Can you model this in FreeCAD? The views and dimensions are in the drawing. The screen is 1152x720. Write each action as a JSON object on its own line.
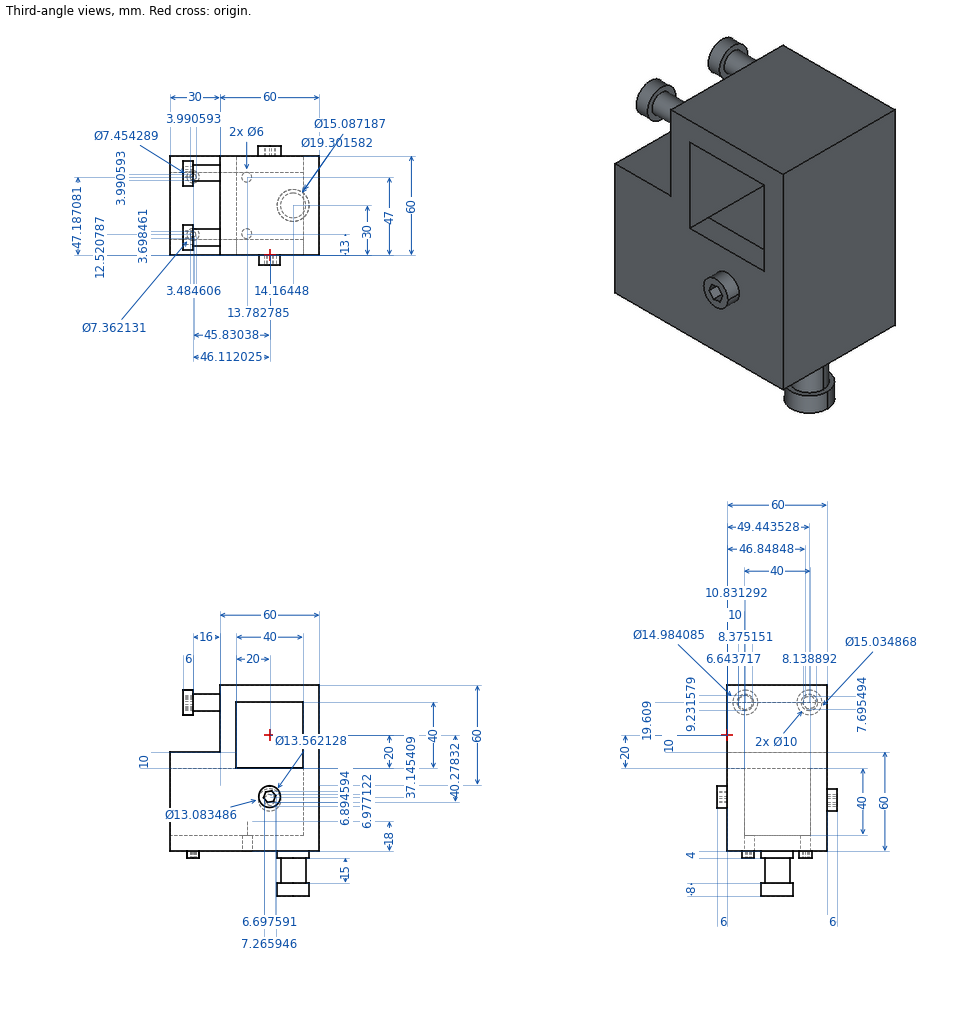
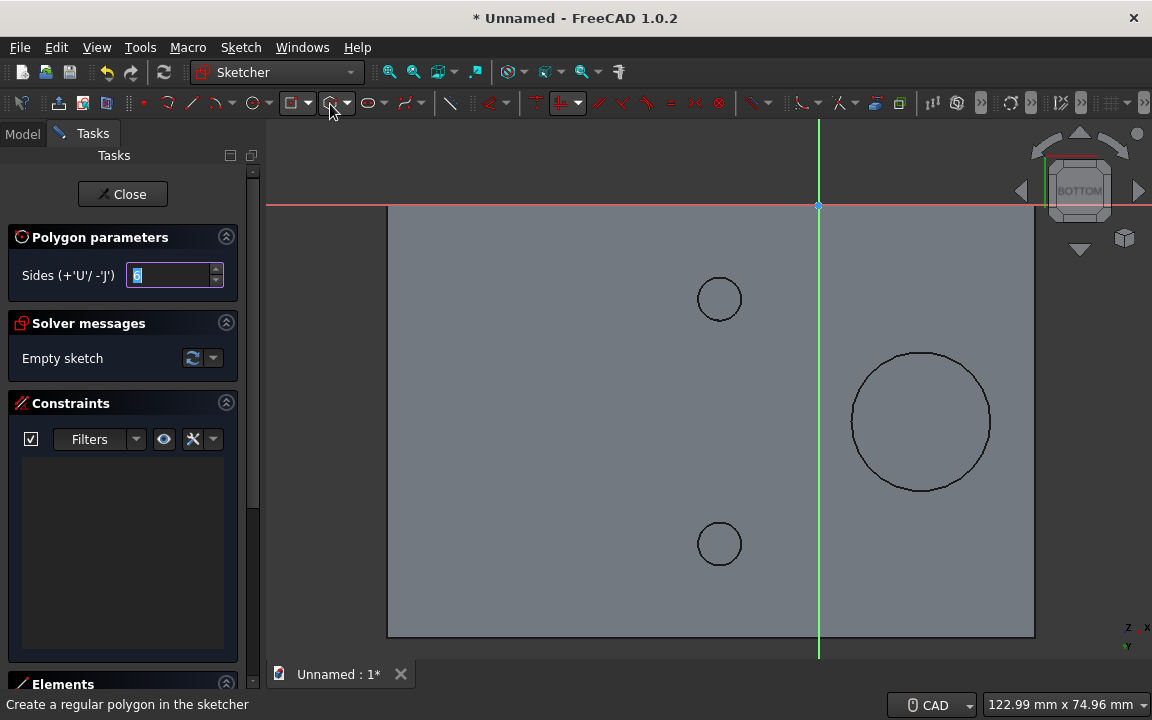
{"action": "scroll", "coordinate": [487, 545], "scroll_direction": "up", "scroll_amount": 4}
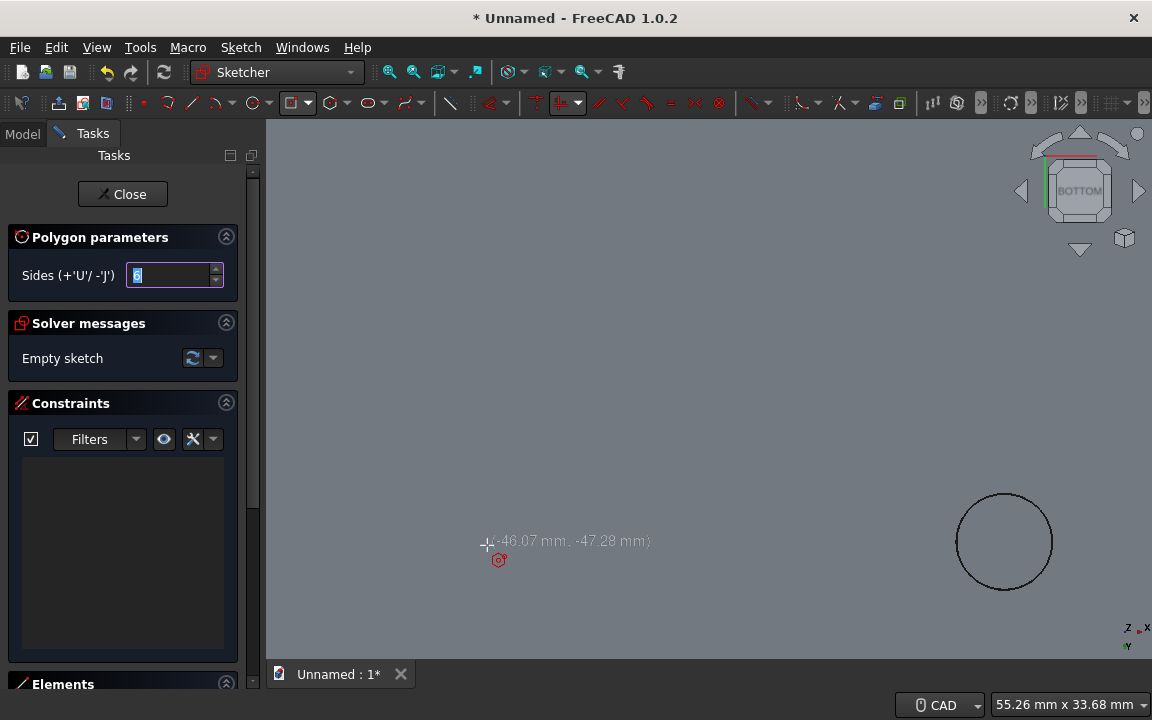
{"action": "left_click", "coordinate": [486, 545]}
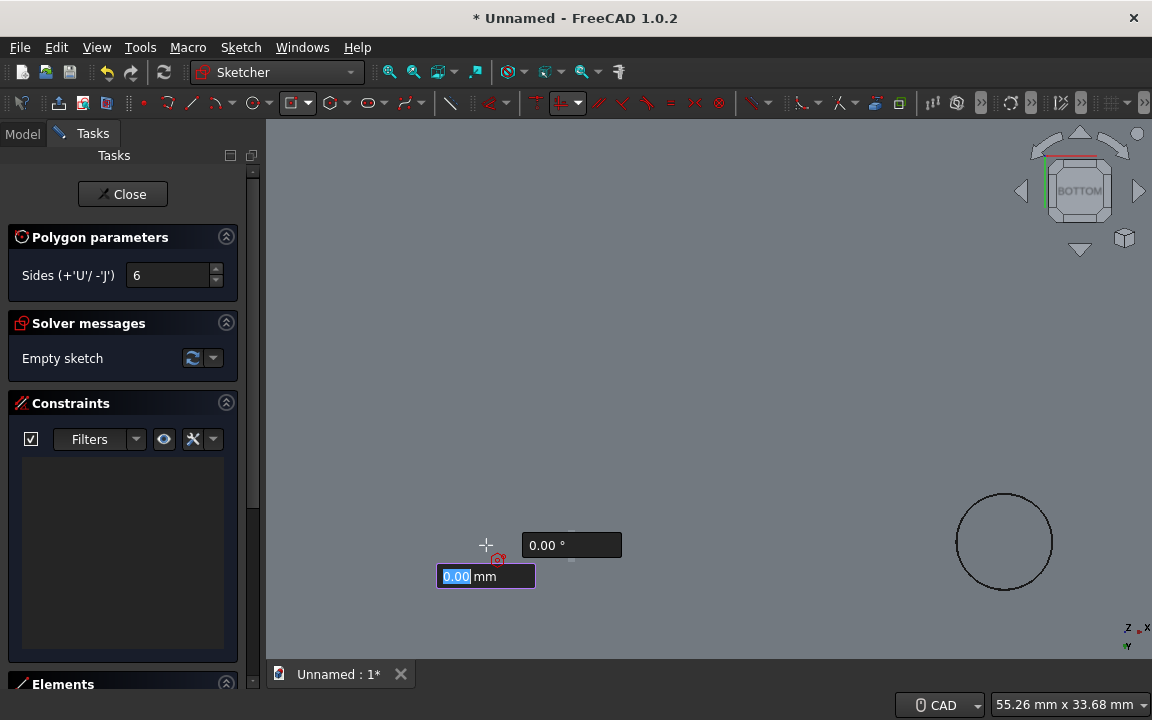
{"action": "left_click", "coordinate": [454, 553]}
{"action": "right_click", "coordinate": [454, 553]}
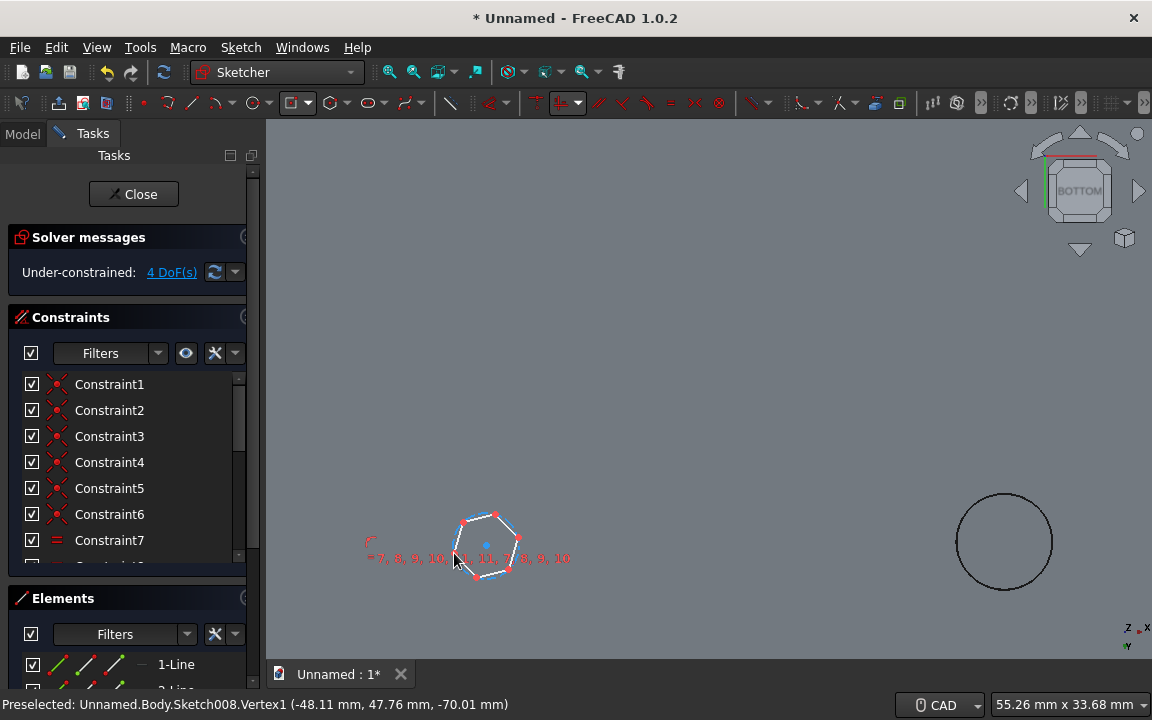
{"action": "left_click", "coordinate": [330, 104]}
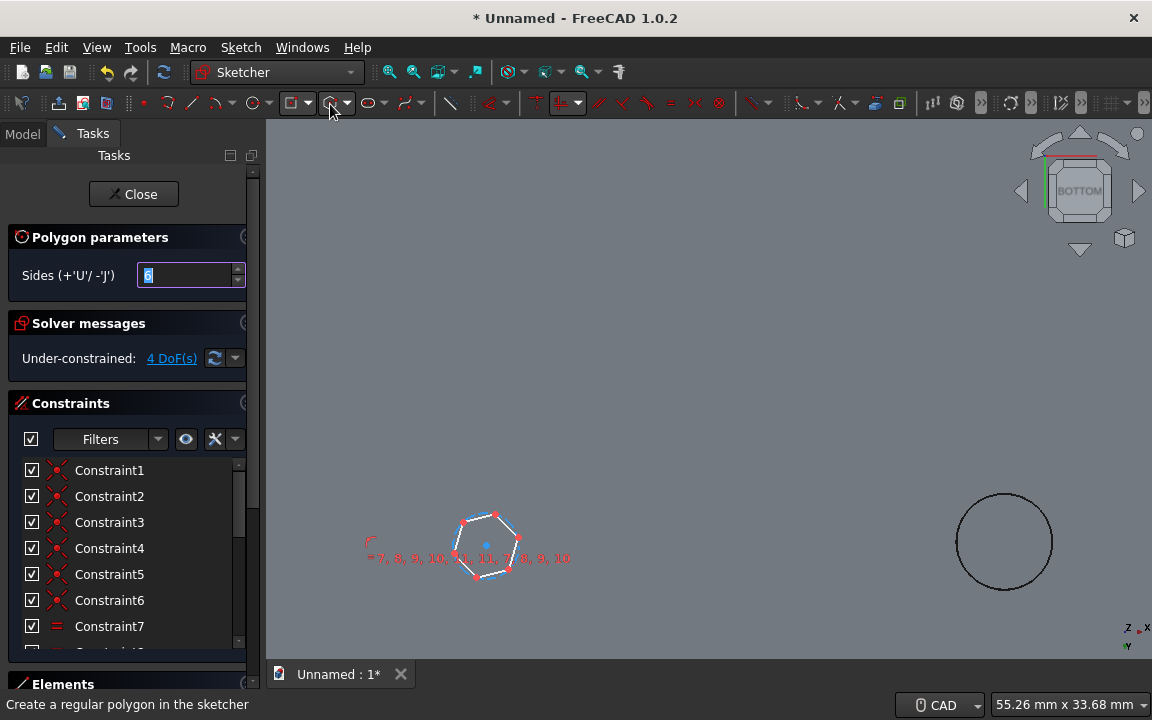
{"action": "scroll", "coordinate": [489, 546], "scroll_direction": "down", "scroll_amount": 4}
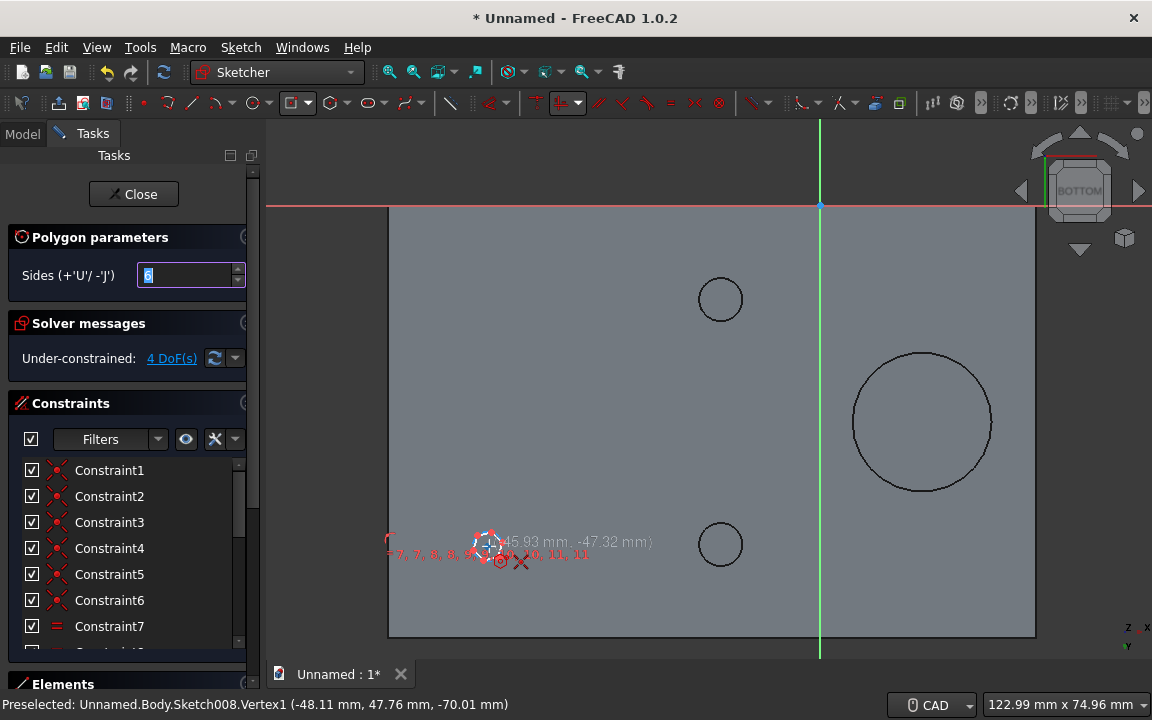
{"action": "scroll", "coordinate": [488, 296], "scroll_direction": "up", "scroll_amount": 5}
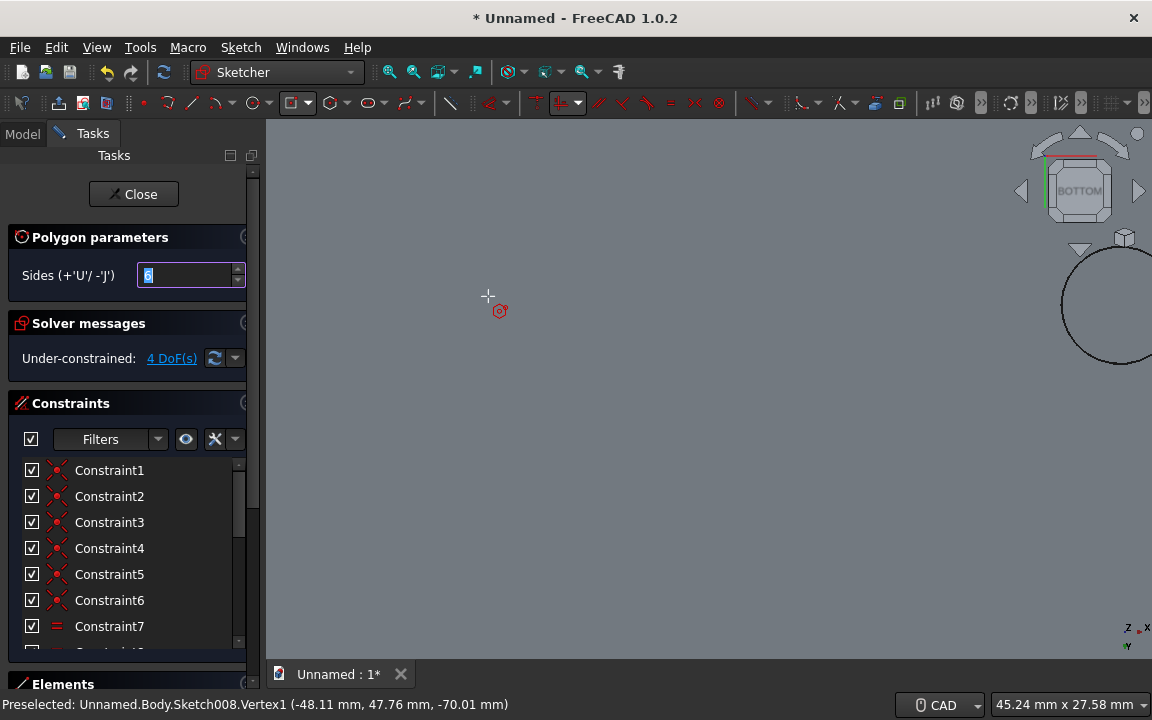
{"action": "left_click", "coordinate": [487, 296]}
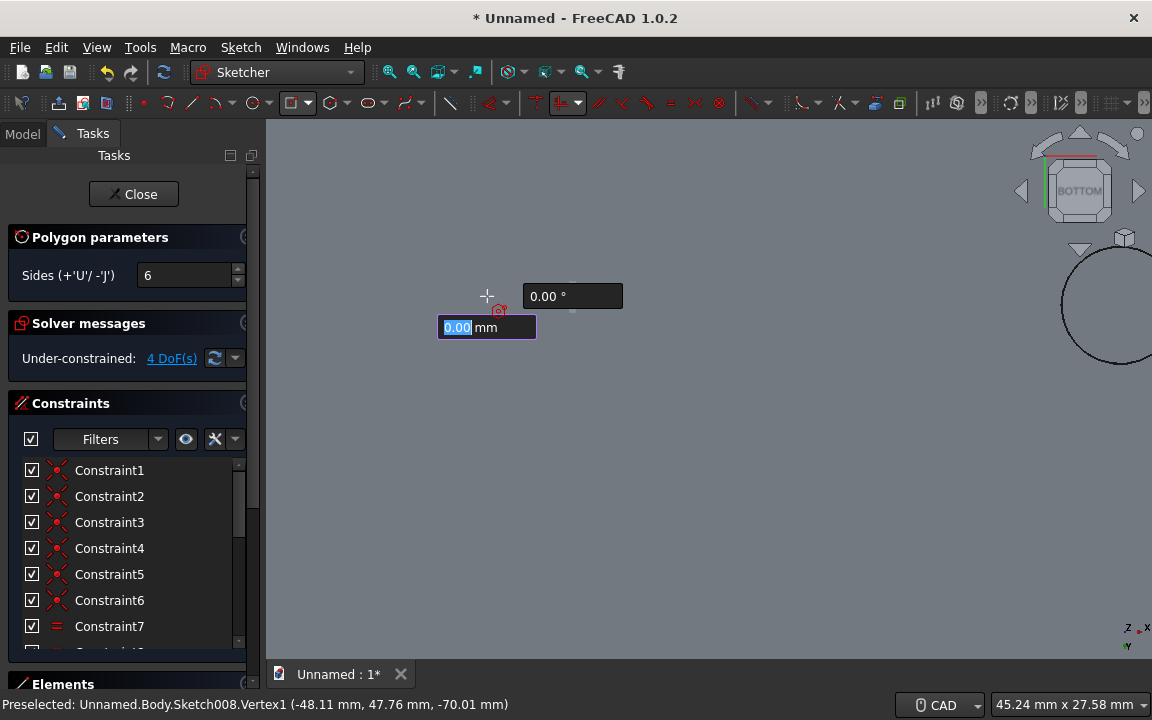
{"action": "left_click", "coordinate": [482, 332]}
{"action": "right_click", "coordinate": [482, 332]}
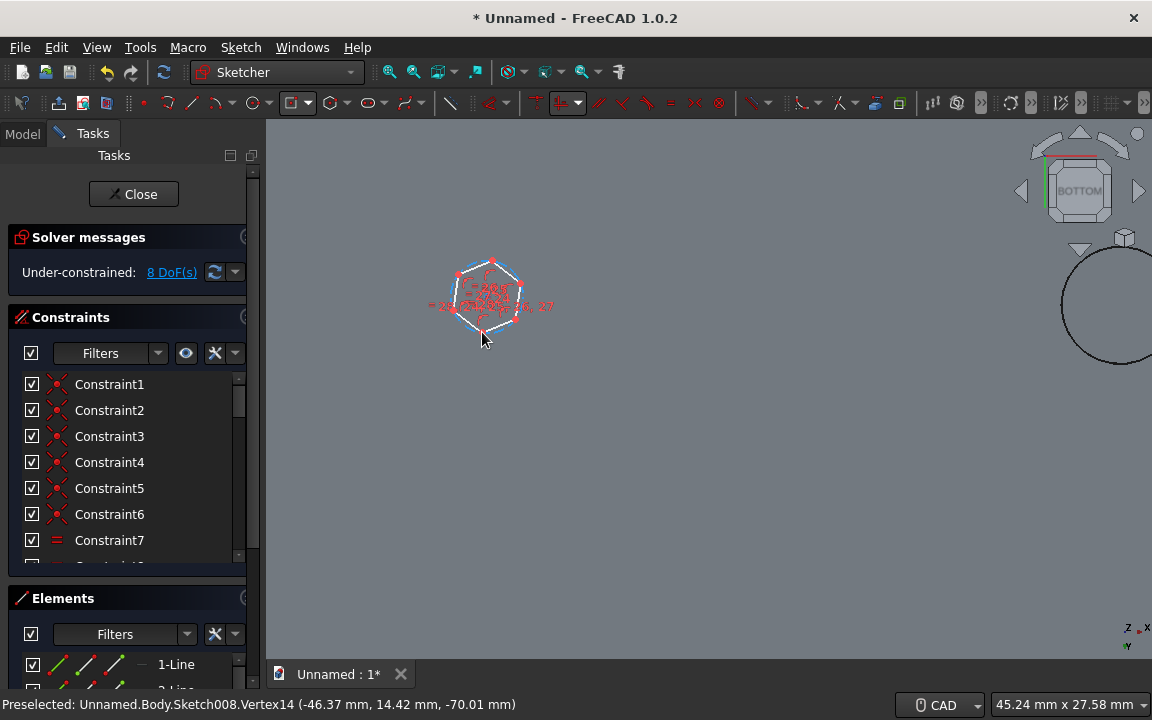
{"action": "left_click", "coordinate": [254, 104]}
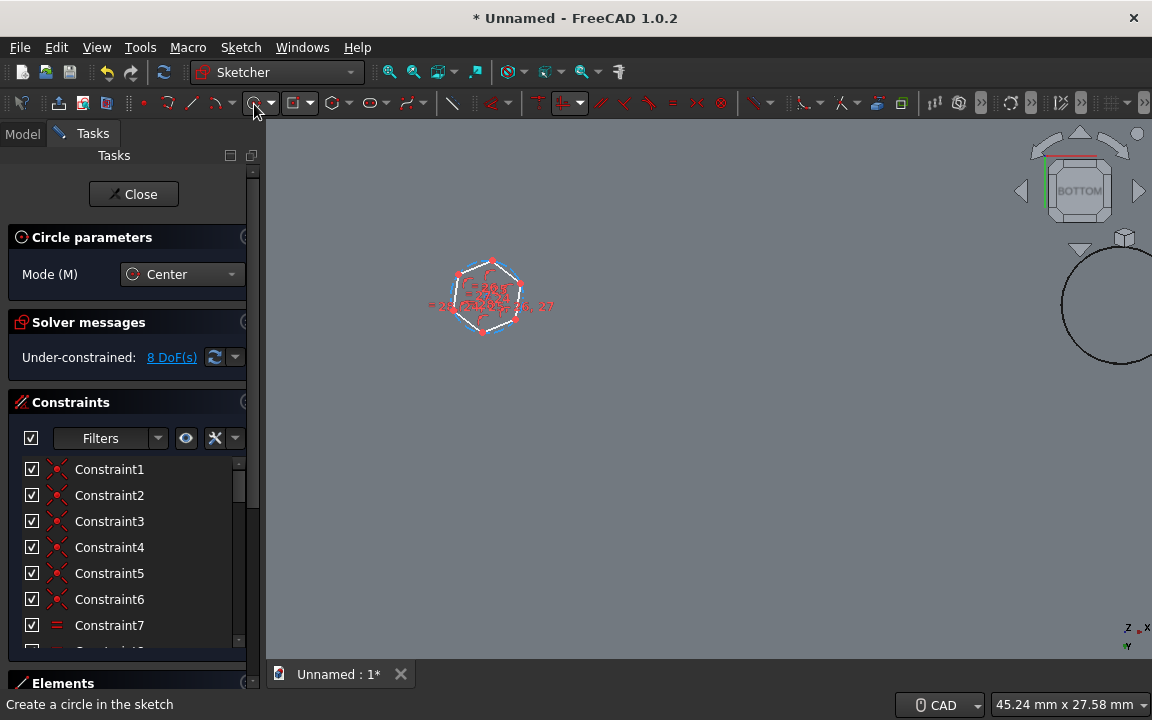
{"action": "scroll", "coordinate": [488, 296], "scroll_direction": "down", "scroll_amount": 5}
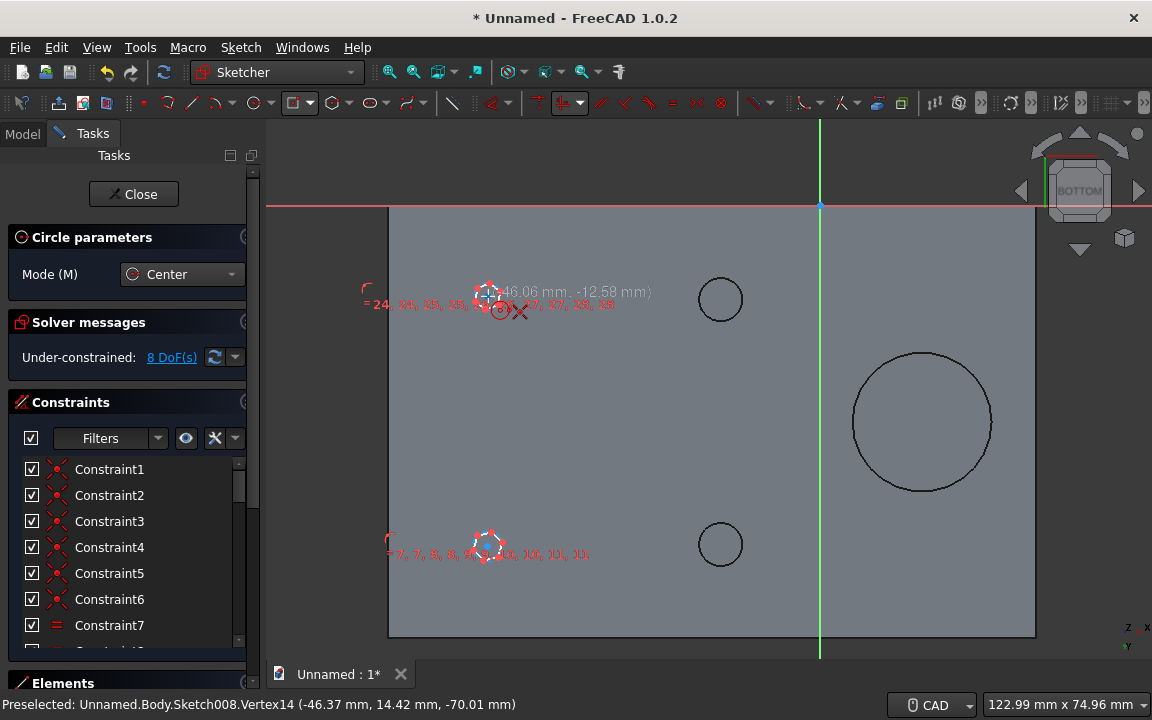
{"action": "scroll", "coordinate": [488, 546], "scroll_direction": "up", "scroll_amount": 2}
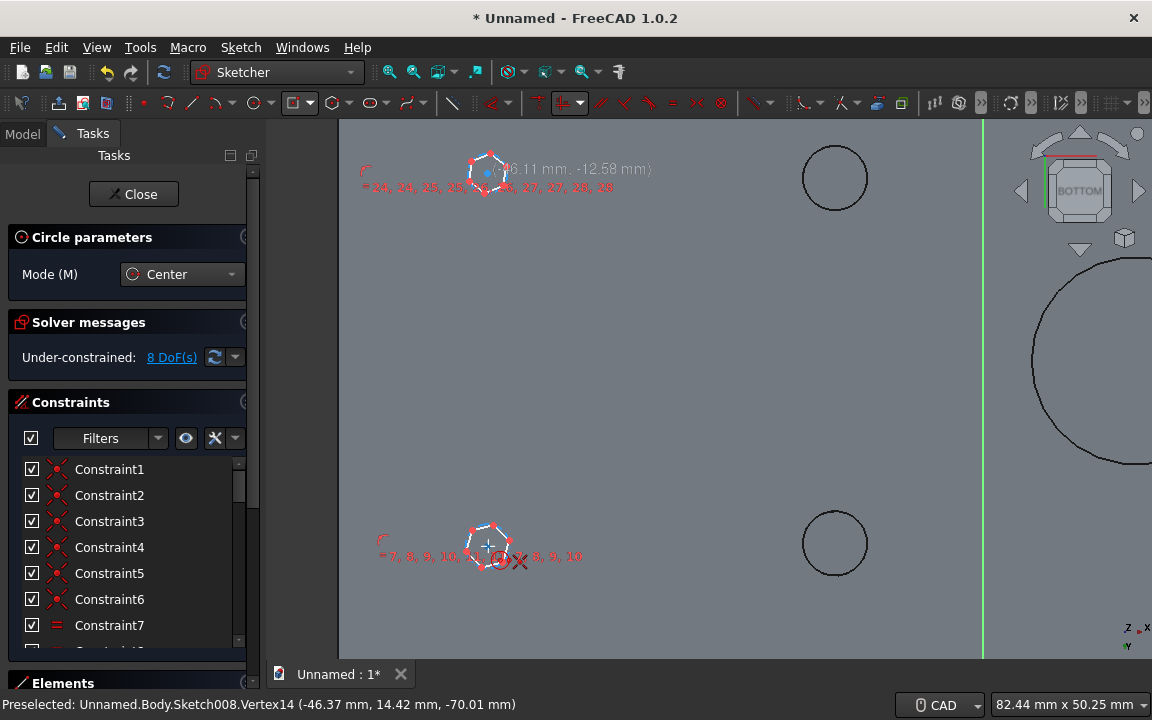
{"action": "left_click", "coordinate": [488, 546]}
{"action": "left_click", "coordinate": [516, 517]}